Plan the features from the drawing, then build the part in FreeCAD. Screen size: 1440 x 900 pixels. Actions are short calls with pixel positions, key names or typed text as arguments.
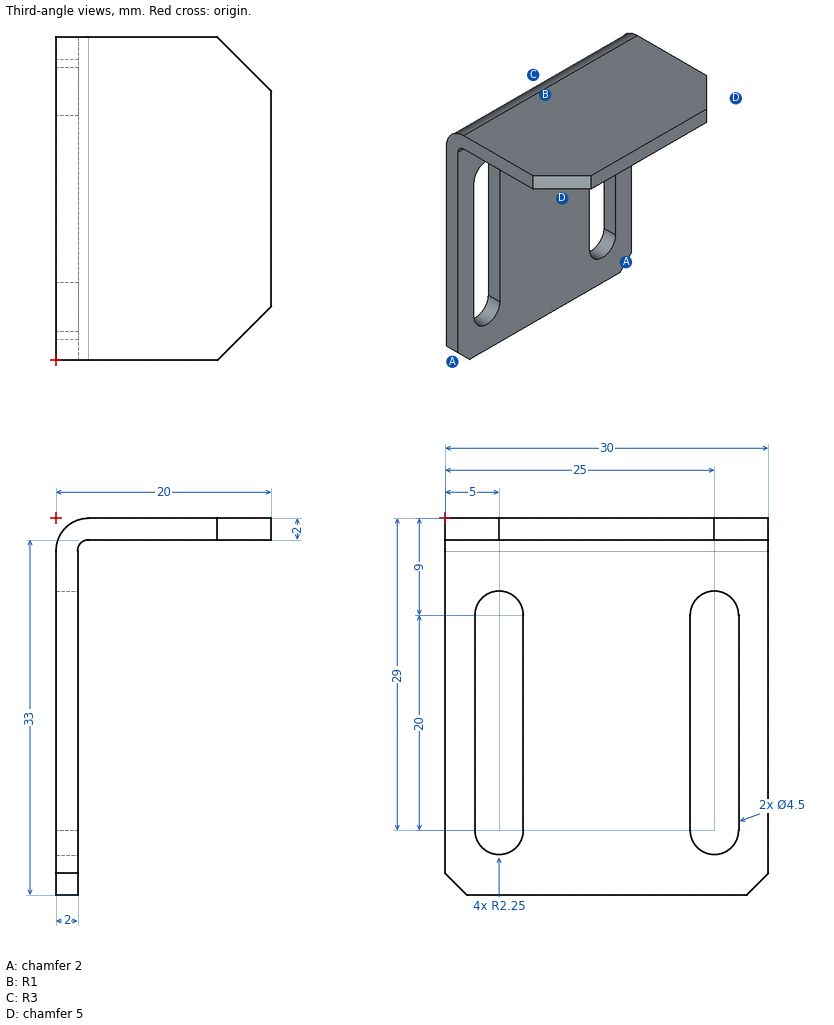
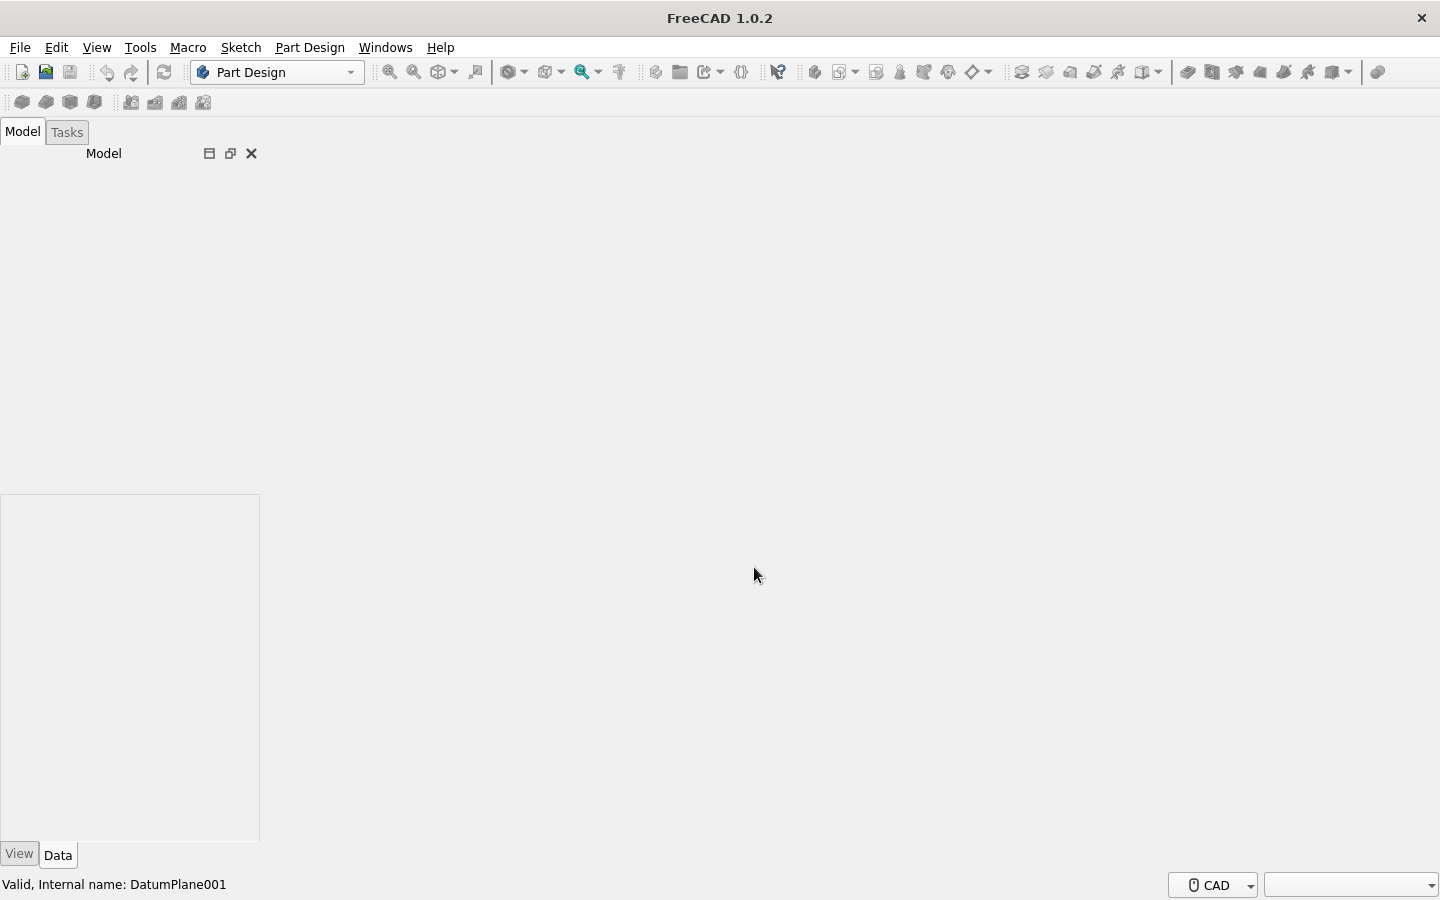
click(22, 72)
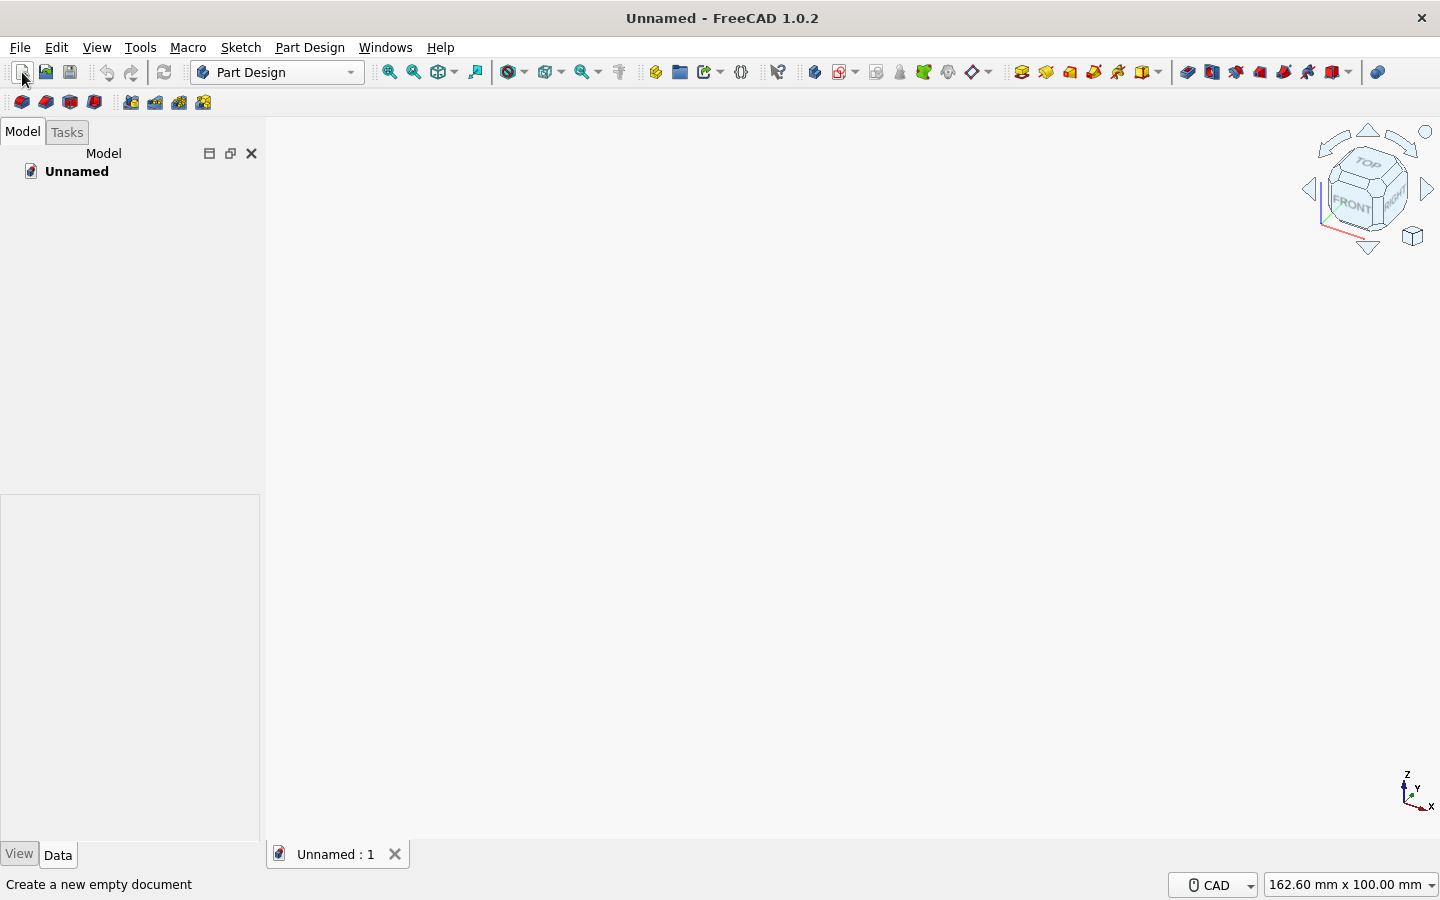
click(840, 72)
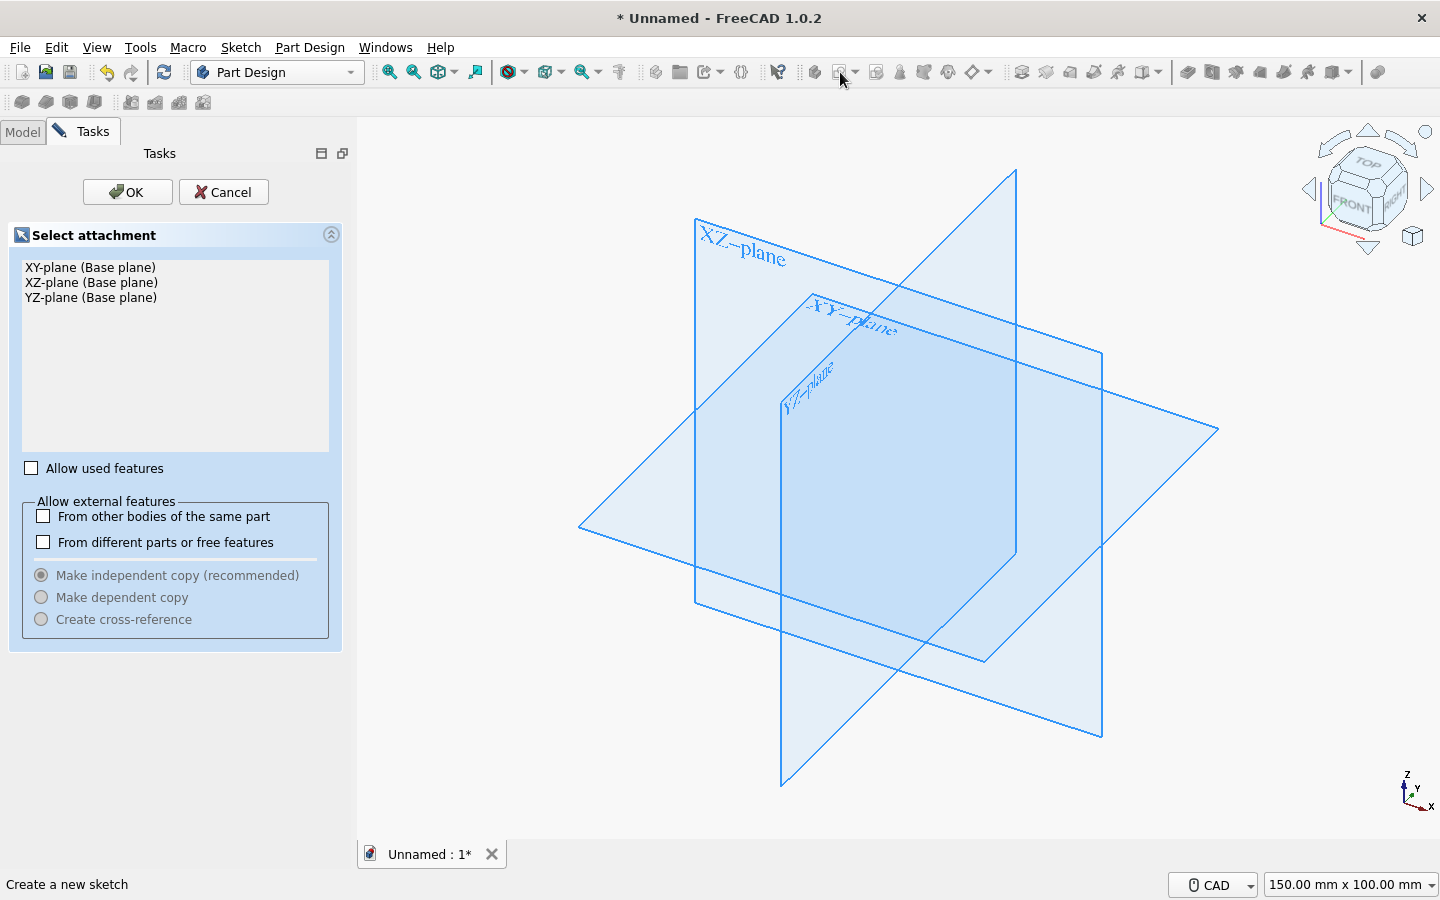
click(82, 282)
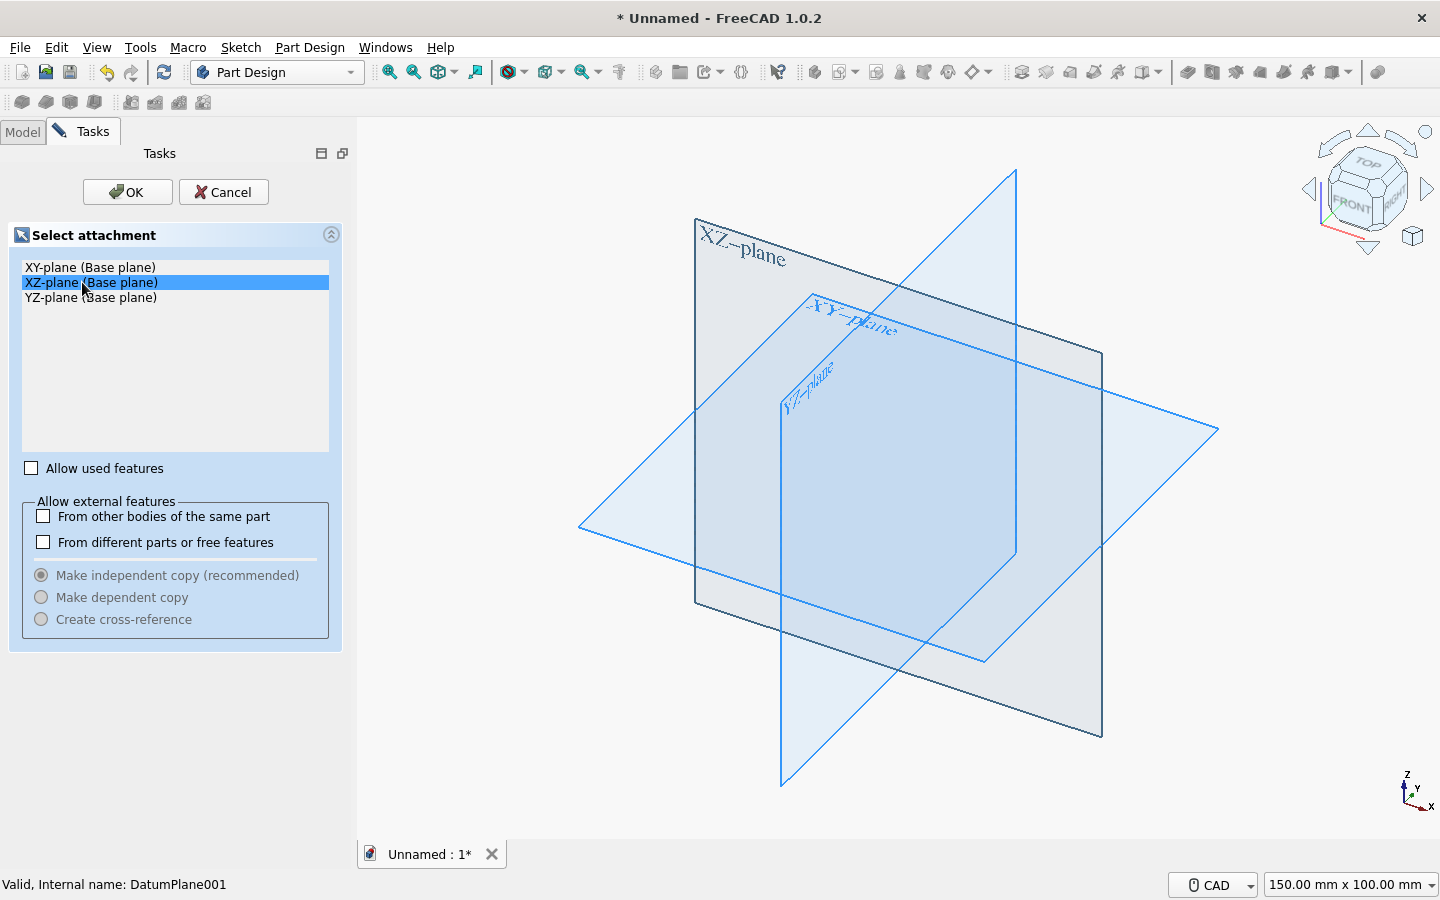
click(128, 192)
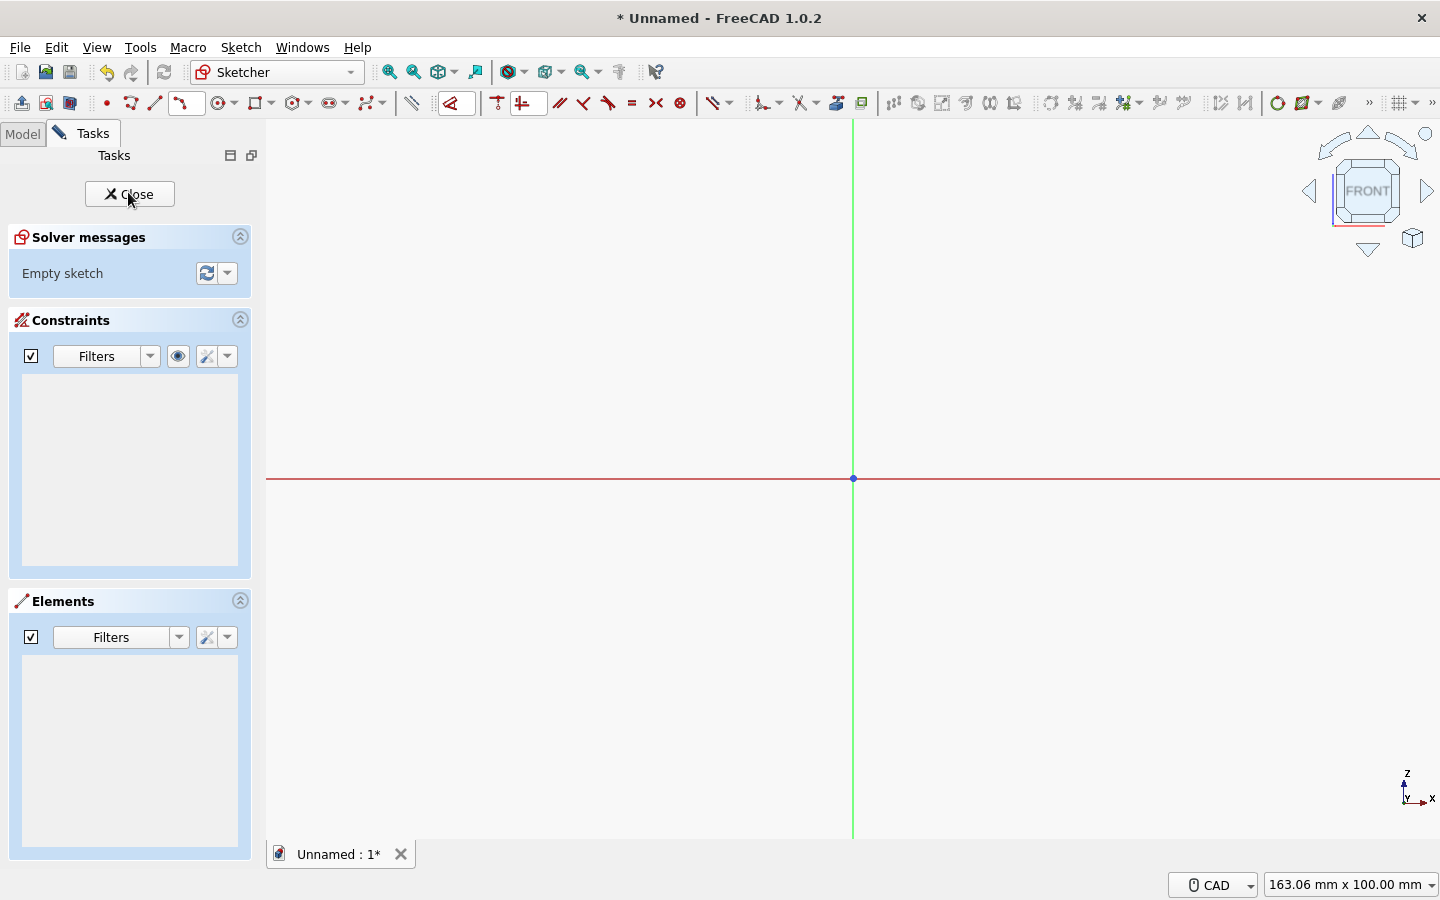
scroll(1096, 758, up, 3)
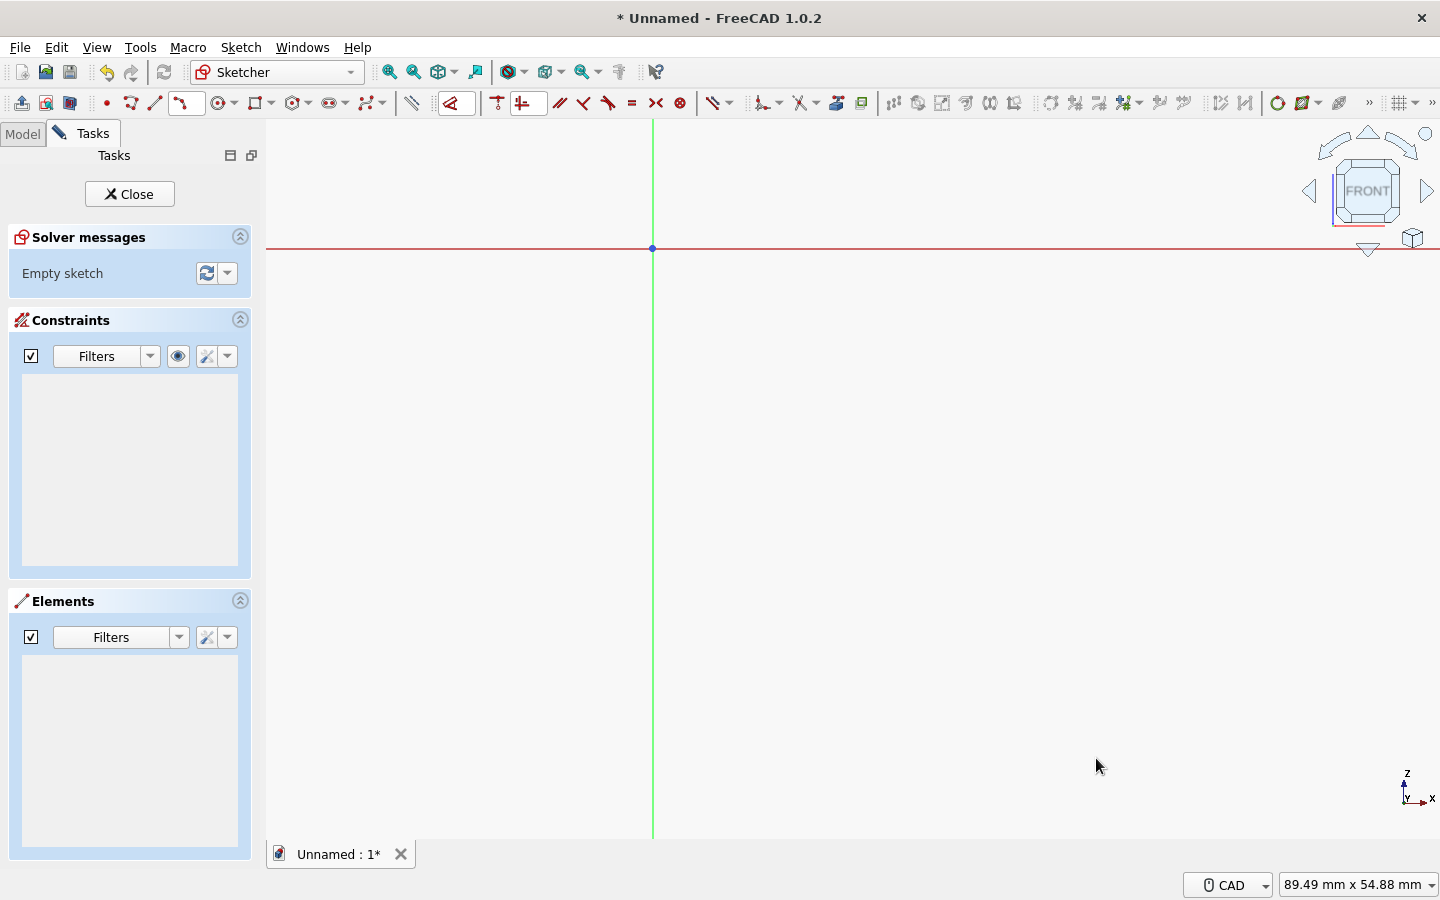
click(132, 104)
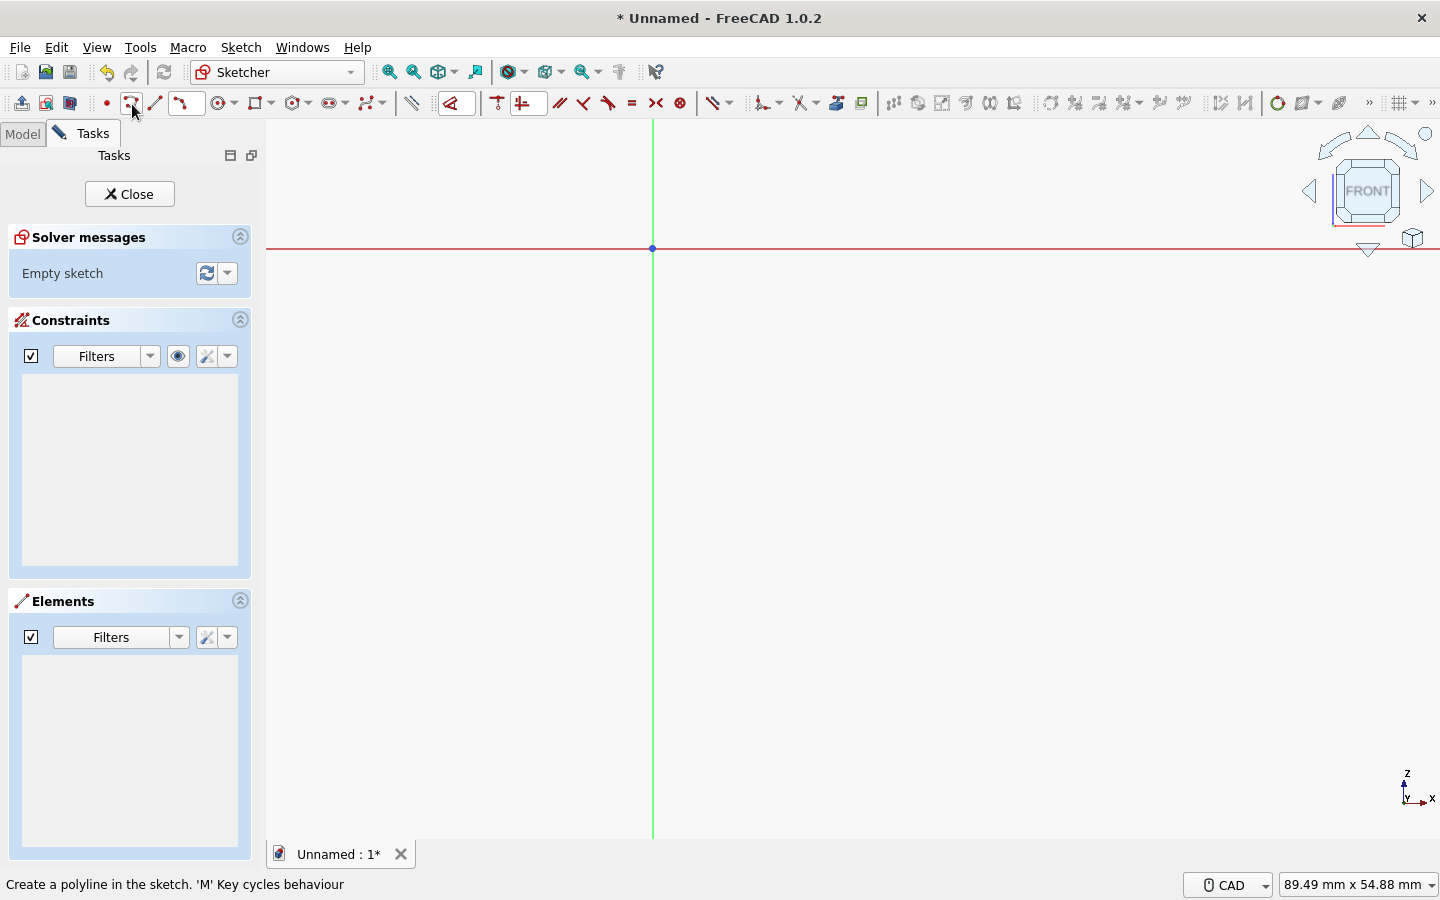
click(653, 249)
click(915, 258)
click(915, 275)
click(679, 275)
click(679, 708)
click(662, 708)
click(653, 249)
key(Escape)
key(Escape)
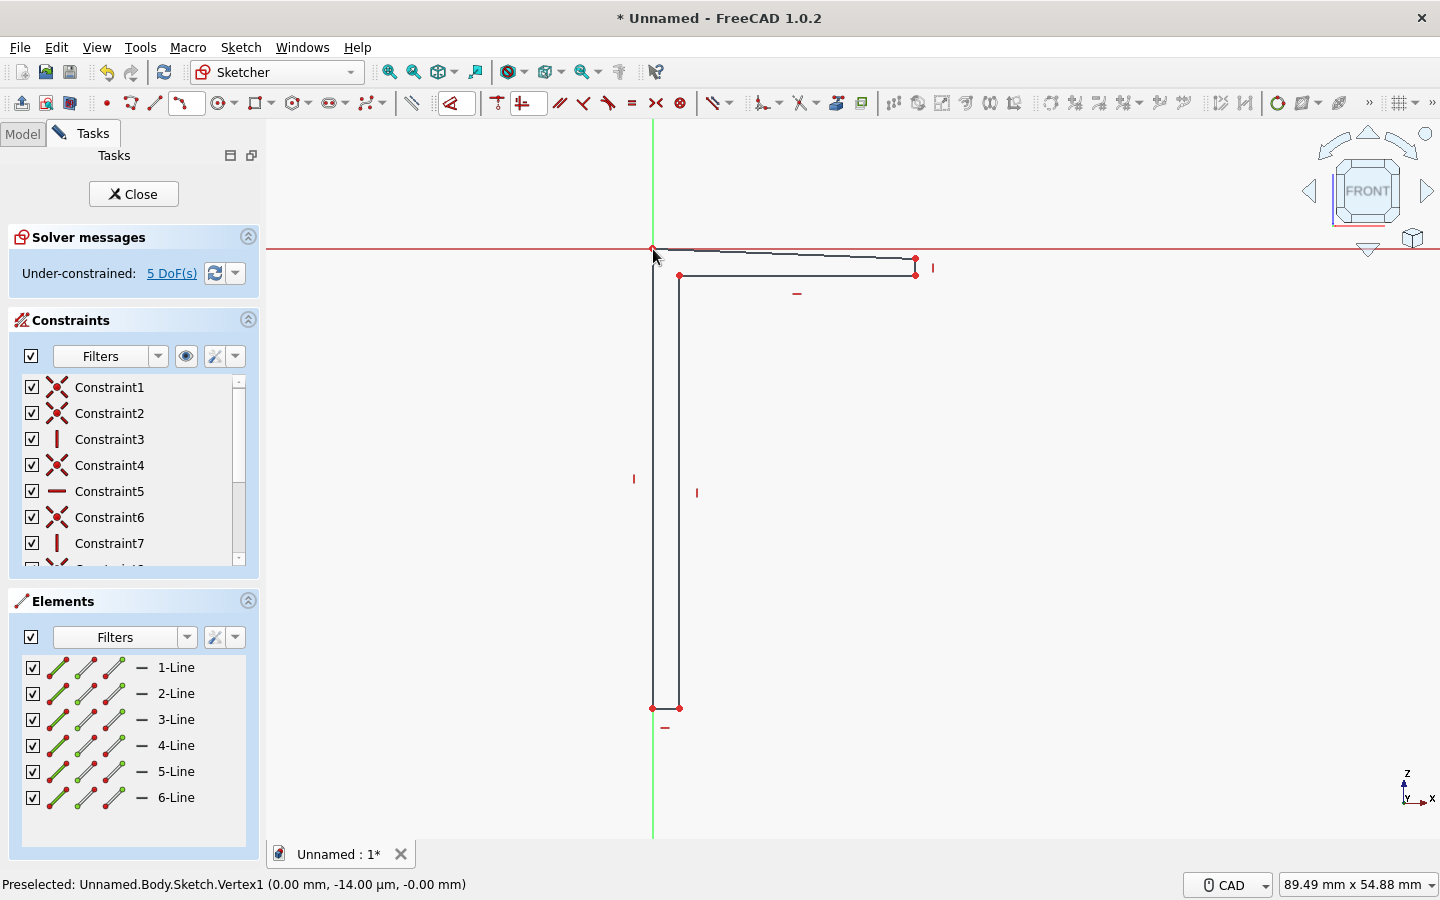
click(731, 252)